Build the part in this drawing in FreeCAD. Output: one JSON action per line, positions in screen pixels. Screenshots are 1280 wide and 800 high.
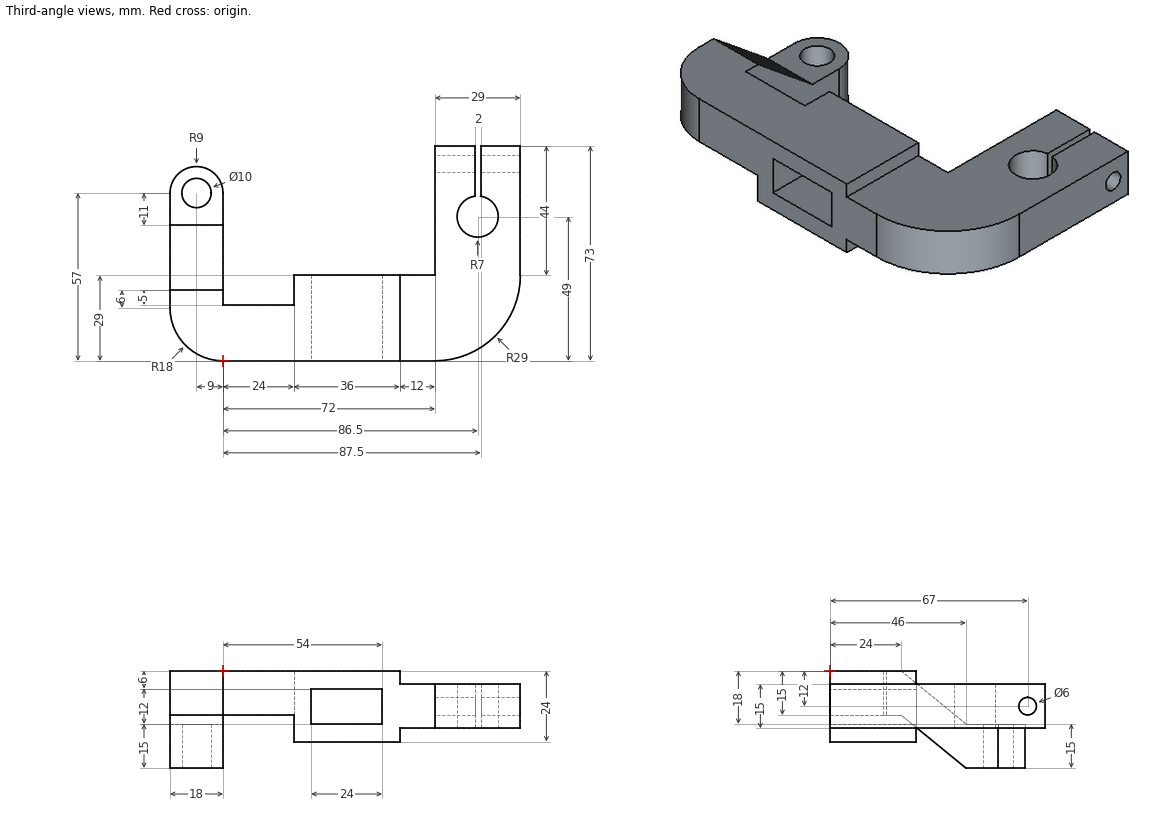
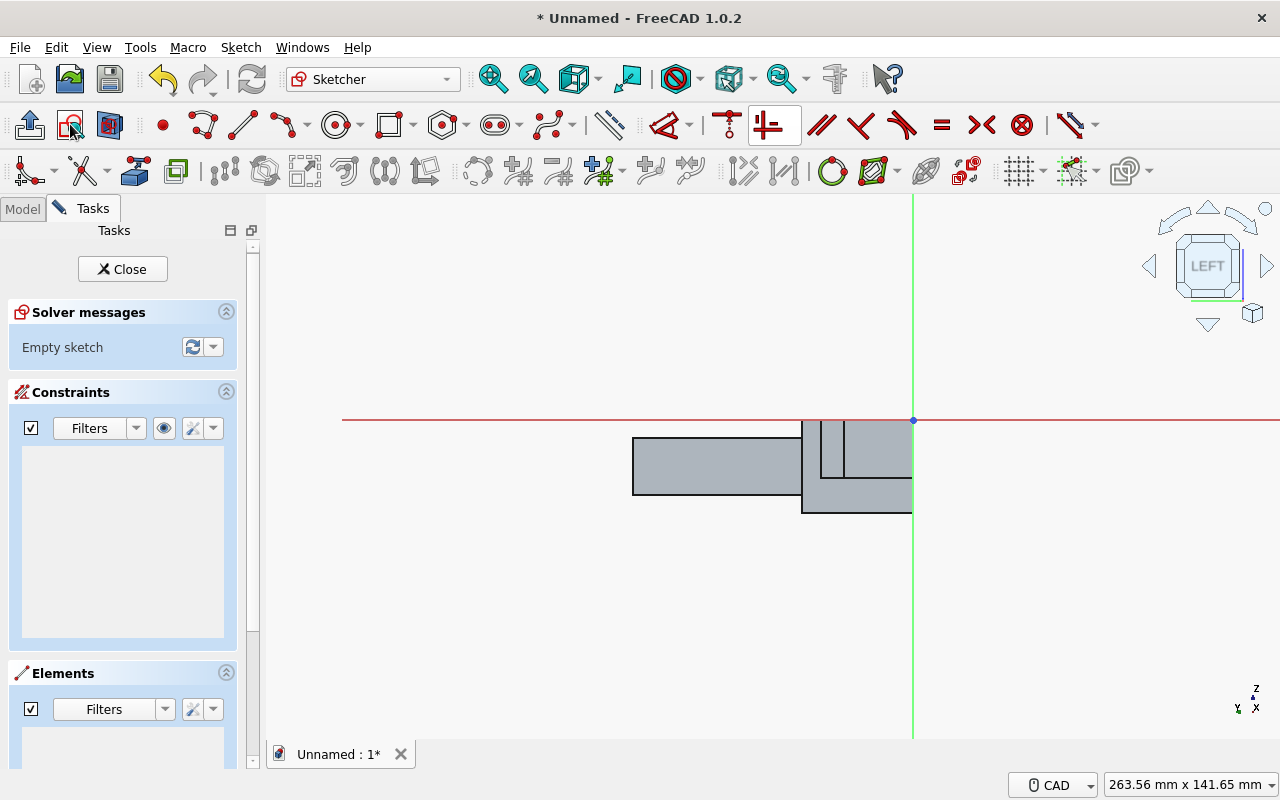
{"action": "scroll", "coordinate": [895, 494], "scroll_direction": "up", "scroll_amount": 5}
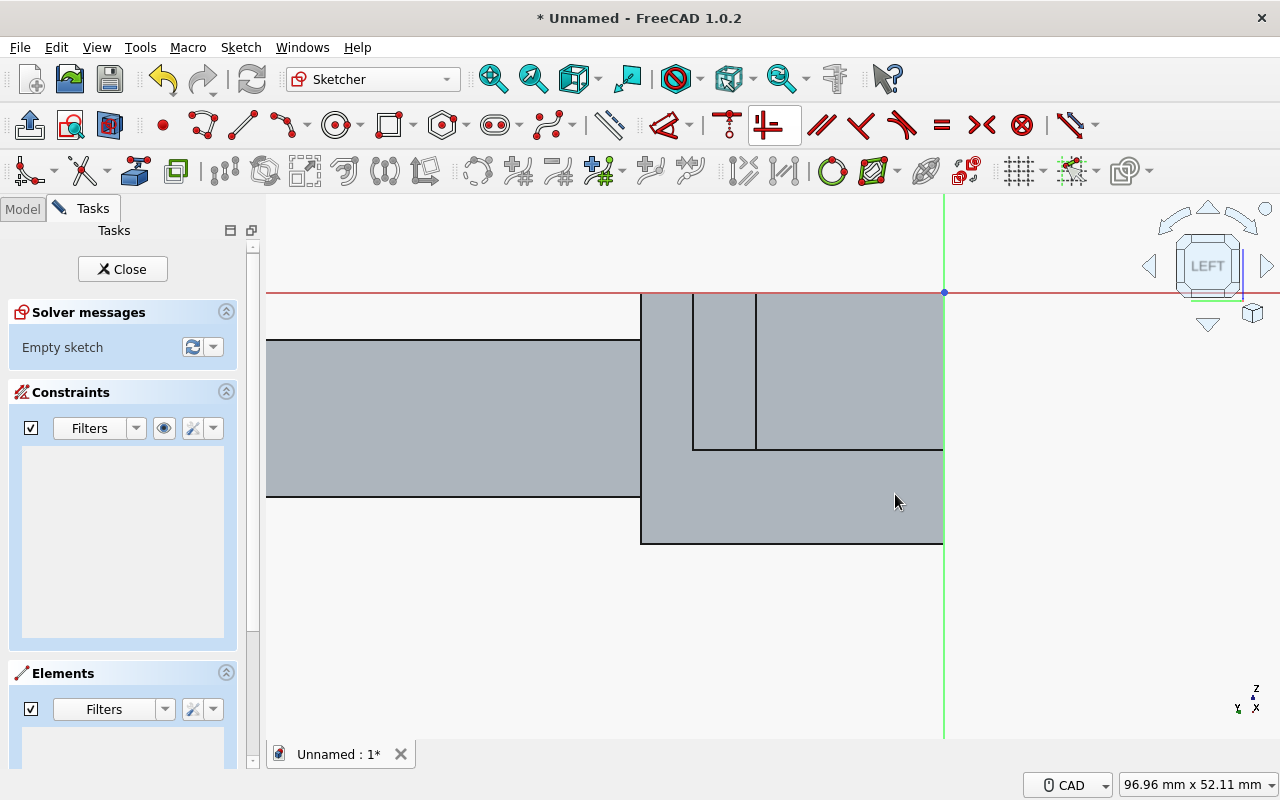
{"action": "left_click", "coordinate": [204, 126]}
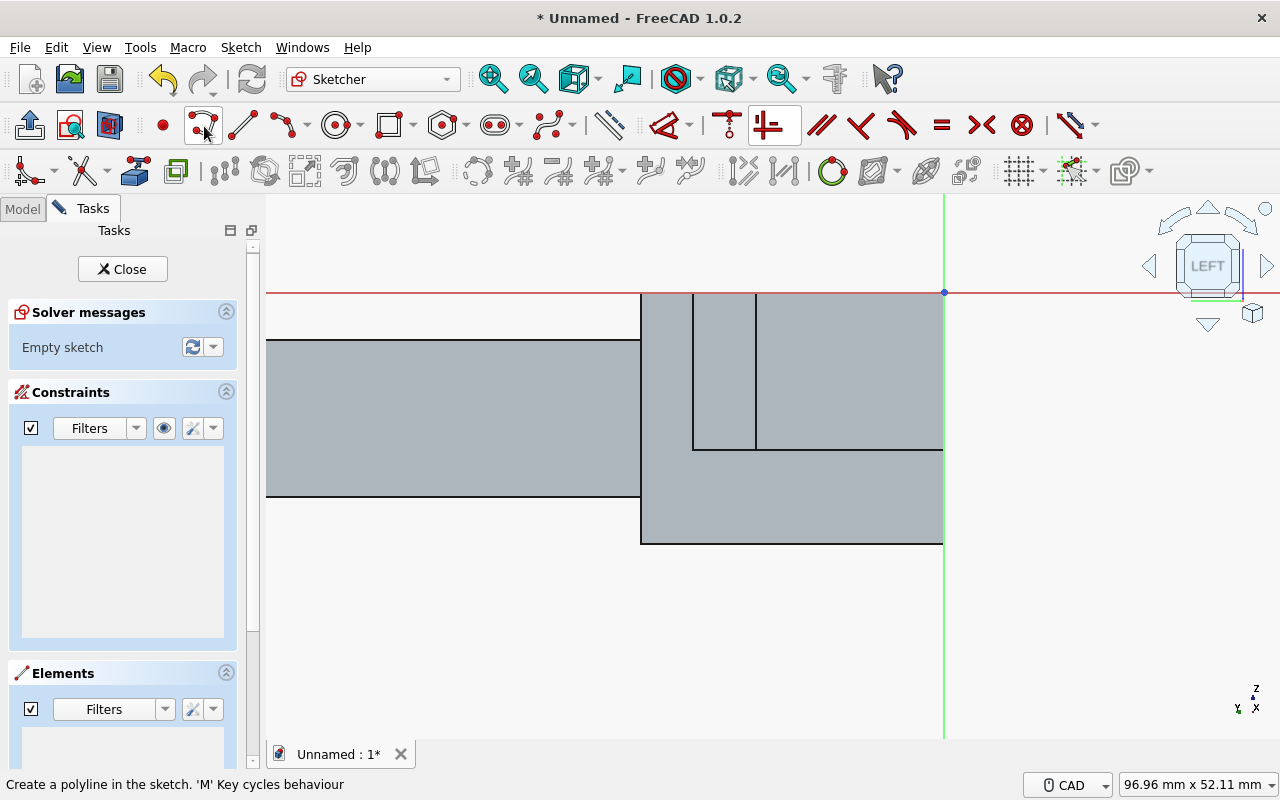
{"action": "left_click", "coordinate": [693, 293]}
{"action": "left_click", "coordinate": [463, 481]}
{"action": "left_click", "coordinate": [463, 638]}
{"action": "left_click", "coordinate": [693, 450]}
{"action": "left_click", "coordinate": [693, 293]}
{"action": "key", "text": "Escape"}
{"action": "key", "text": "Escape"}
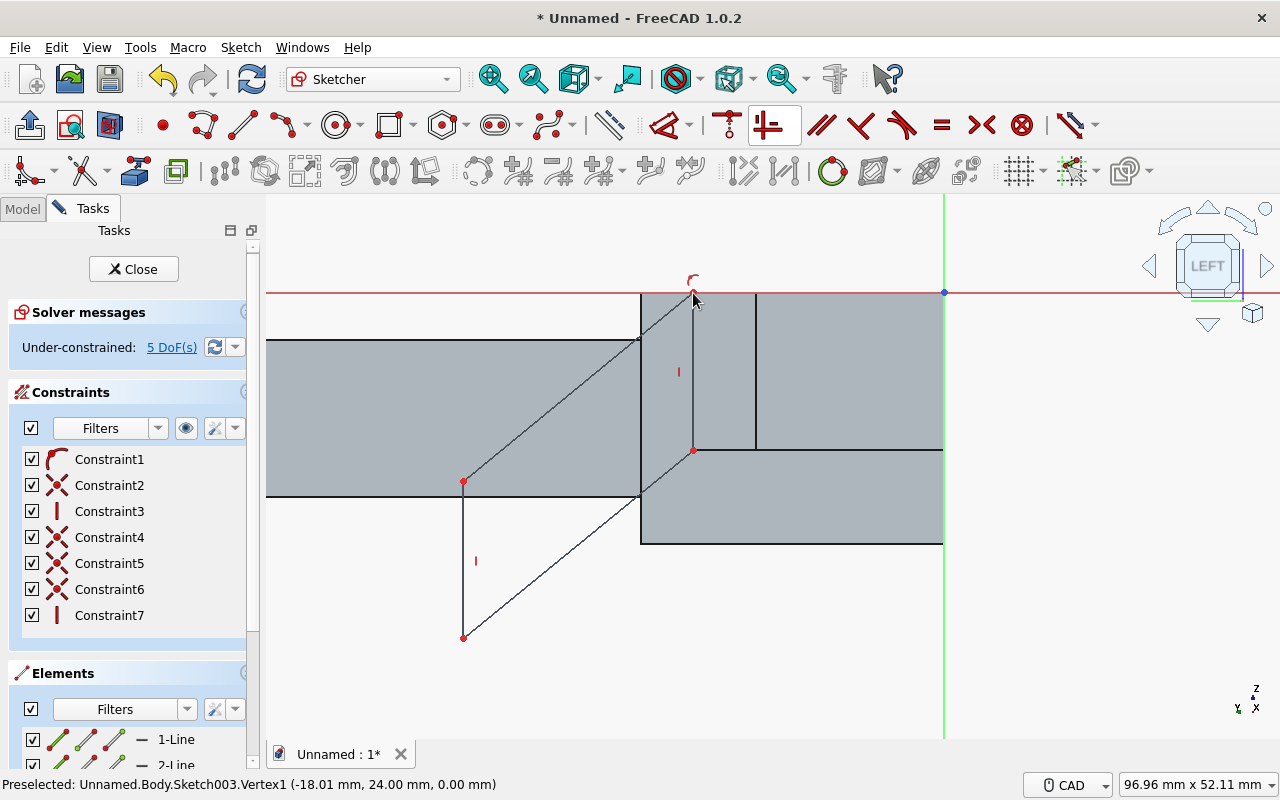
{"action": "key", "text": "d"}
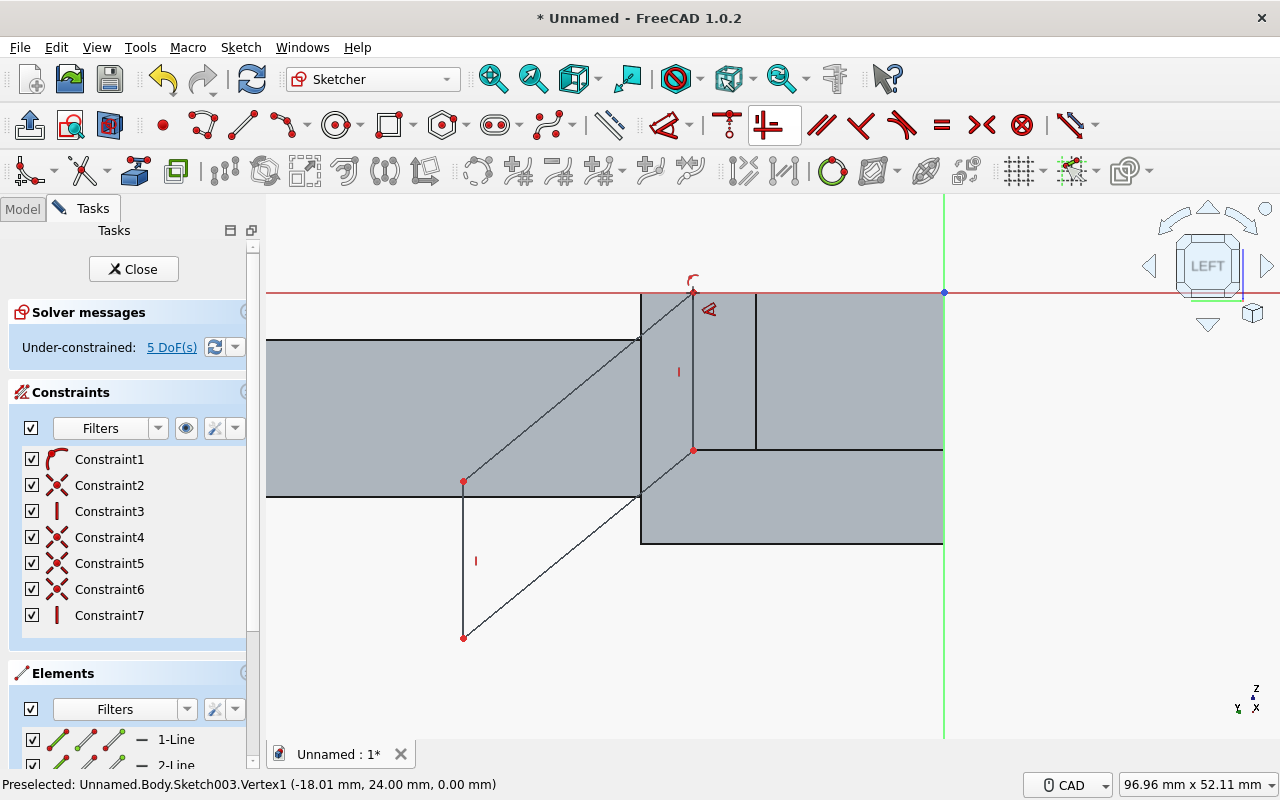
{"action": "left_click", "coordinate": [463, 529]}
{"action": "left_click", "coordinate": [429, 560]}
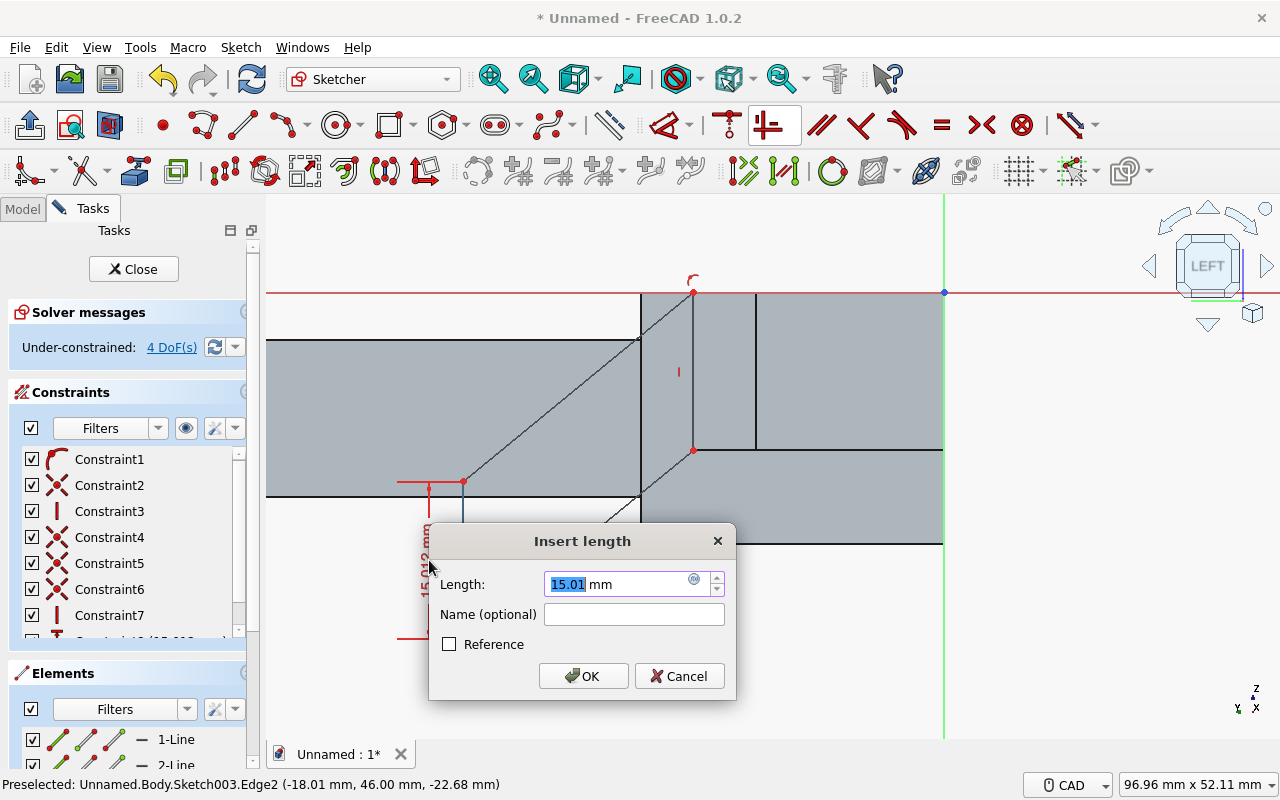
{"action": "type", "text": "15"}
{"action": "key", "text": "Return"}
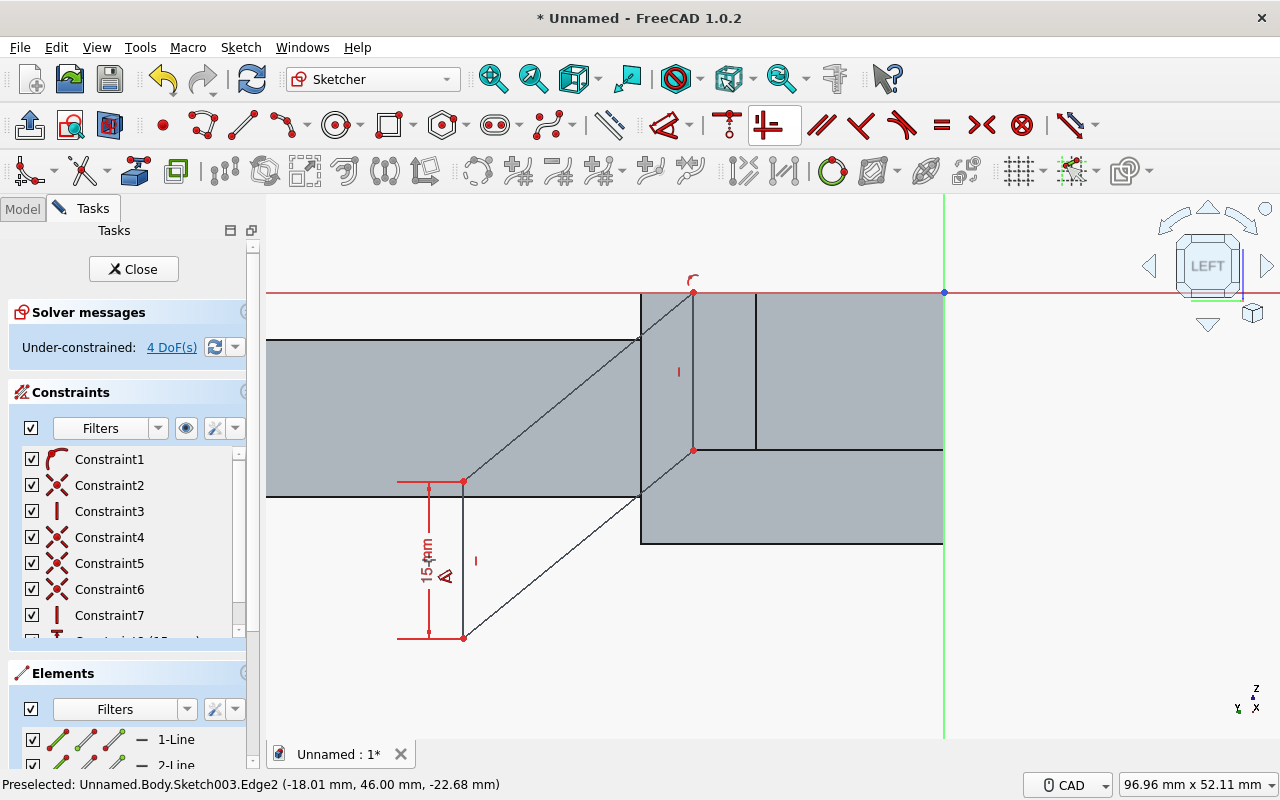
{"action": "left_click", "coordinate": [693, 404]}
{"action": "left_click", "coordinate": [659, 372]}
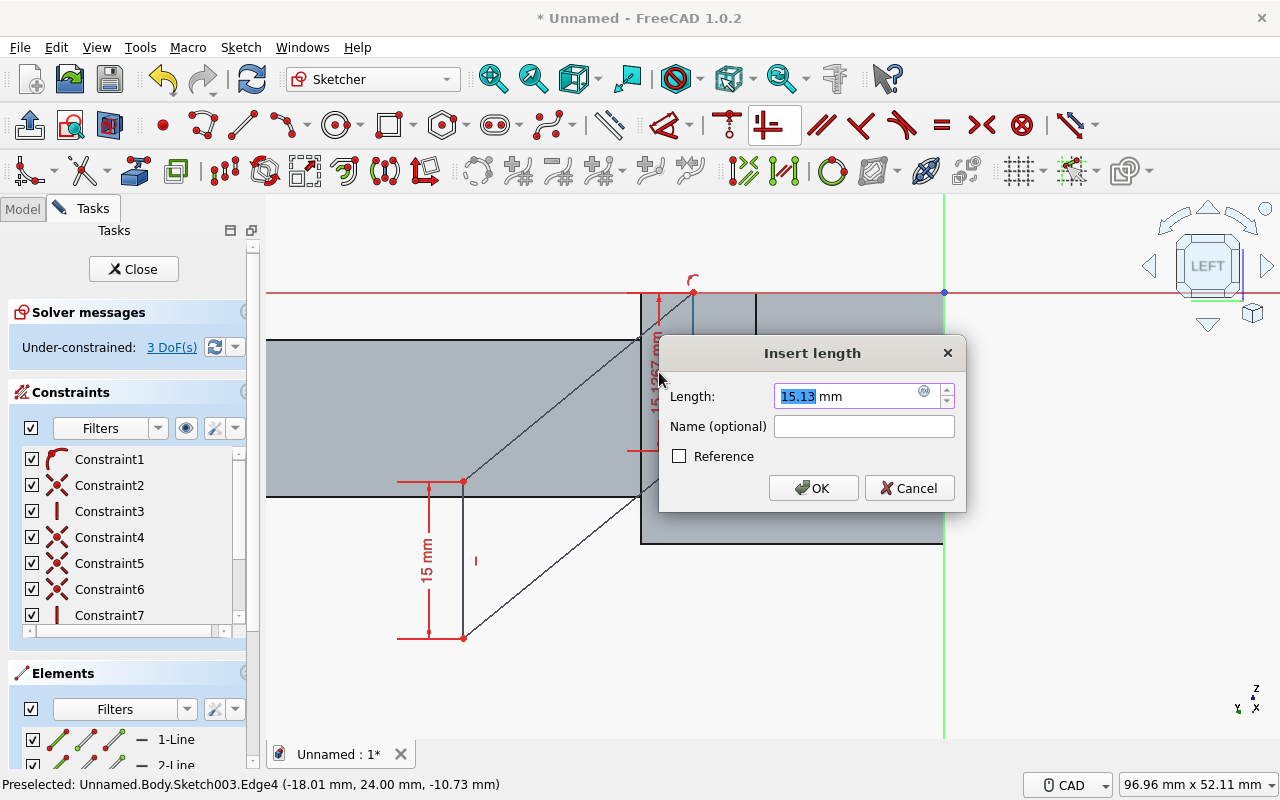
{"action": "type", "text": "15"}
{"action": "key", "text": "Return"}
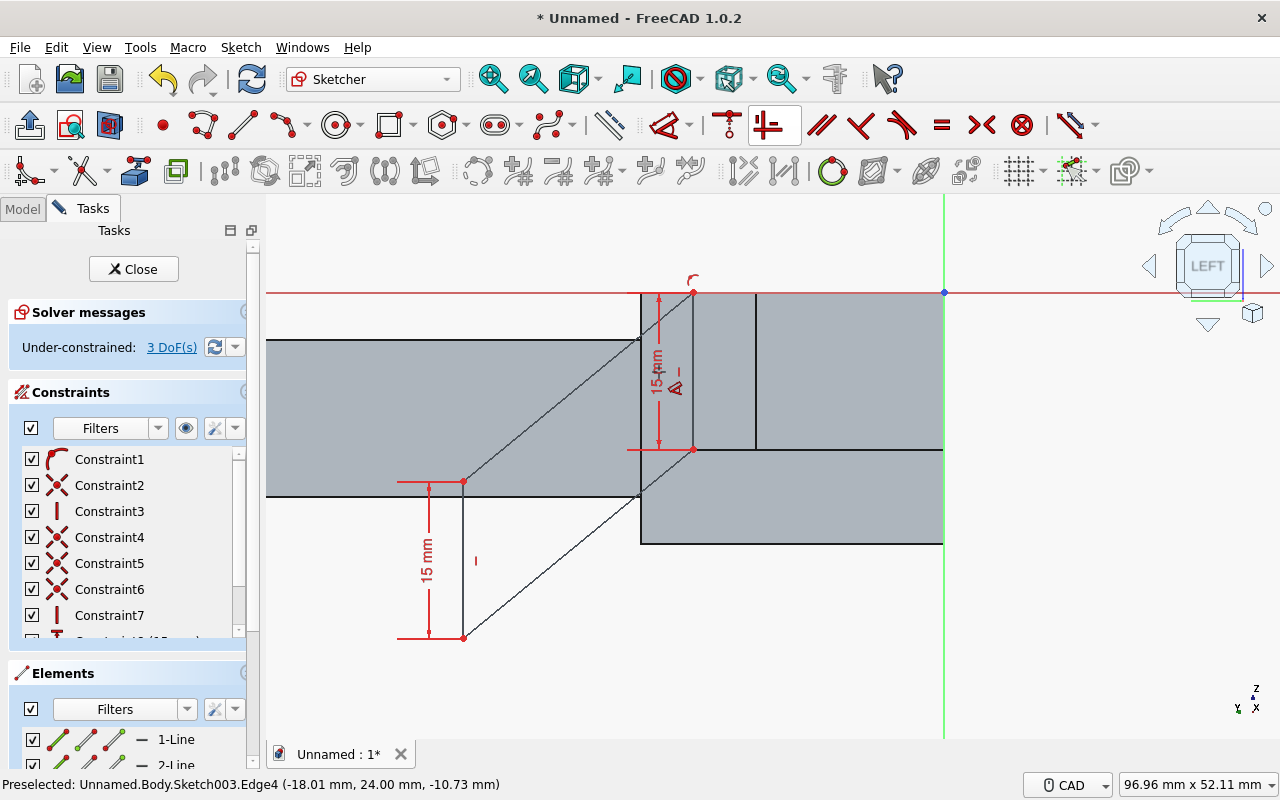
{"action": "left_click", "coordinate": [693, 293]}
{"action": "left_click", "coordinate": [819, 259]}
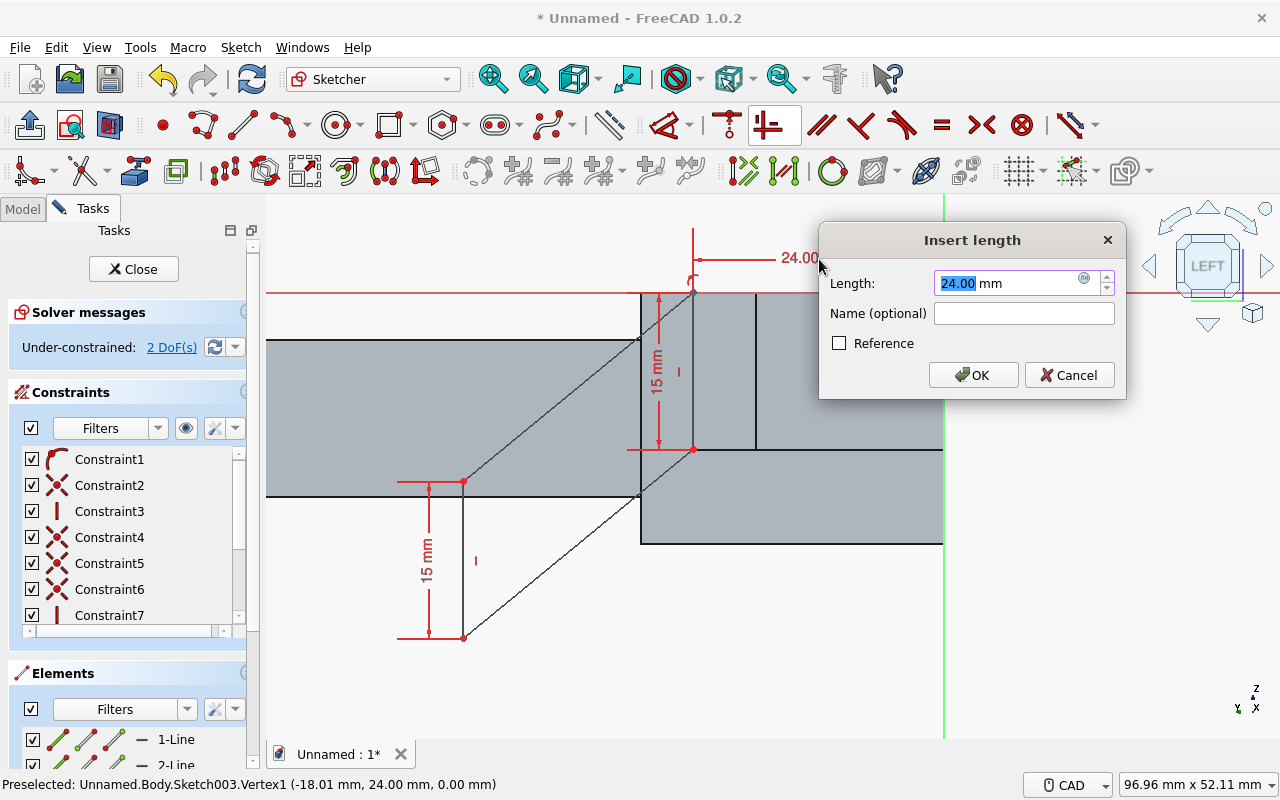
{"action": "type", "text": "24"}
{"action": "key", "text": "Return"}